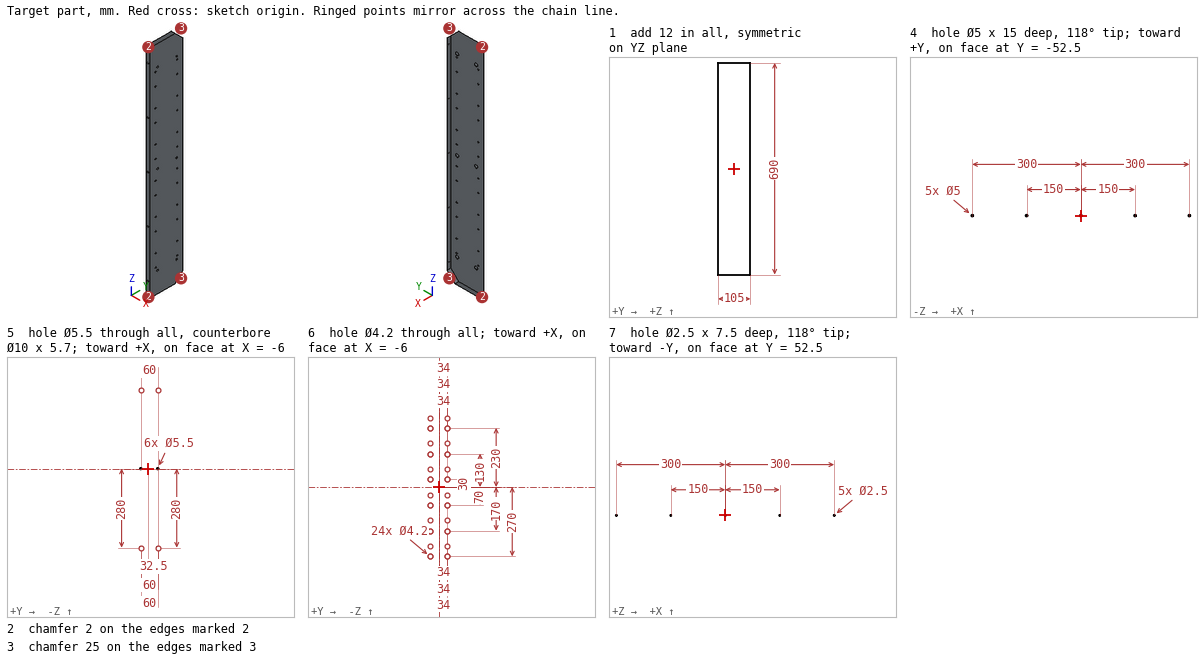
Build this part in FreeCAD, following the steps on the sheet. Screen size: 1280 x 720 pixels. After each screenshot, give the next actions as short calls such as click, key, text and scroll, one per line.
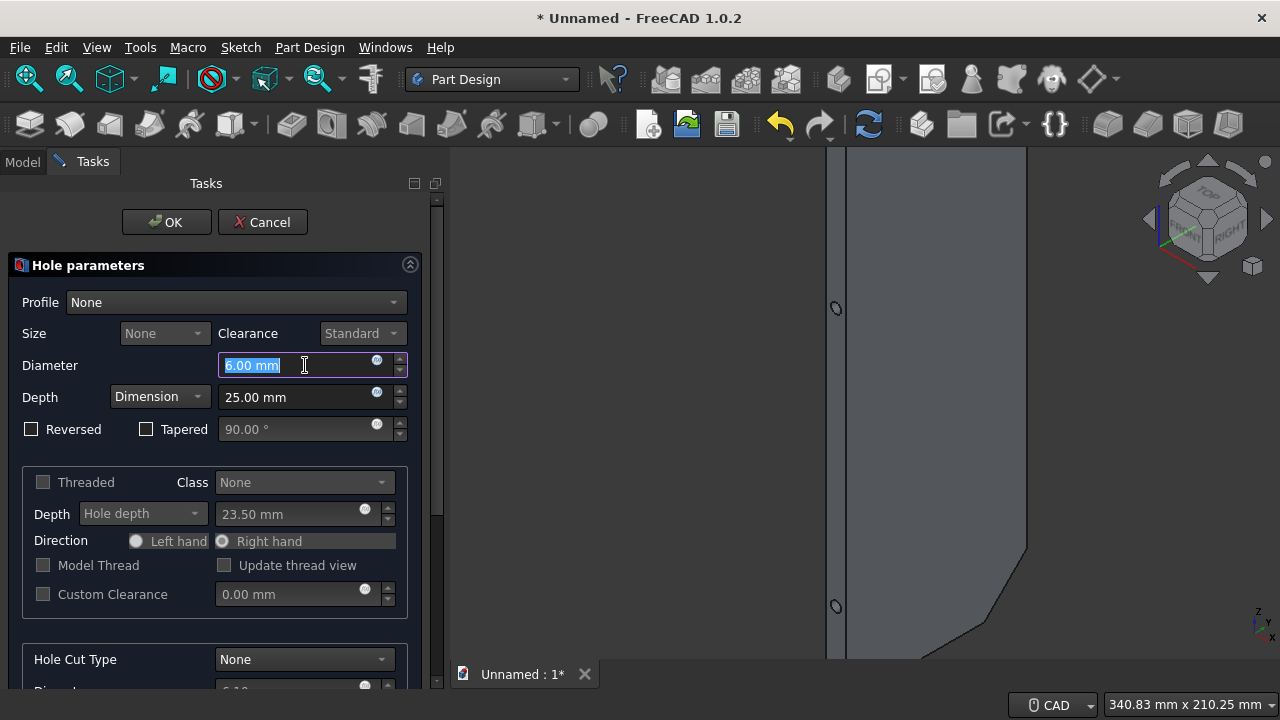
text(5)
key(Tab)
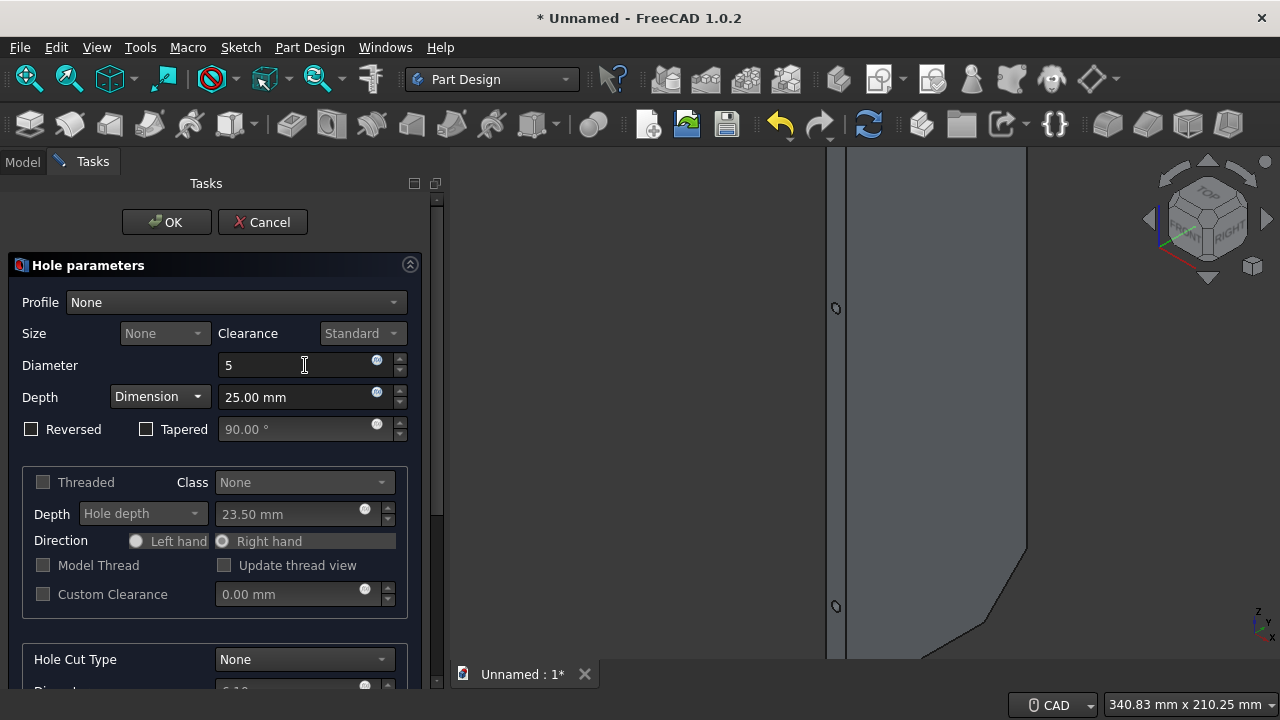
triple_click(305, 397)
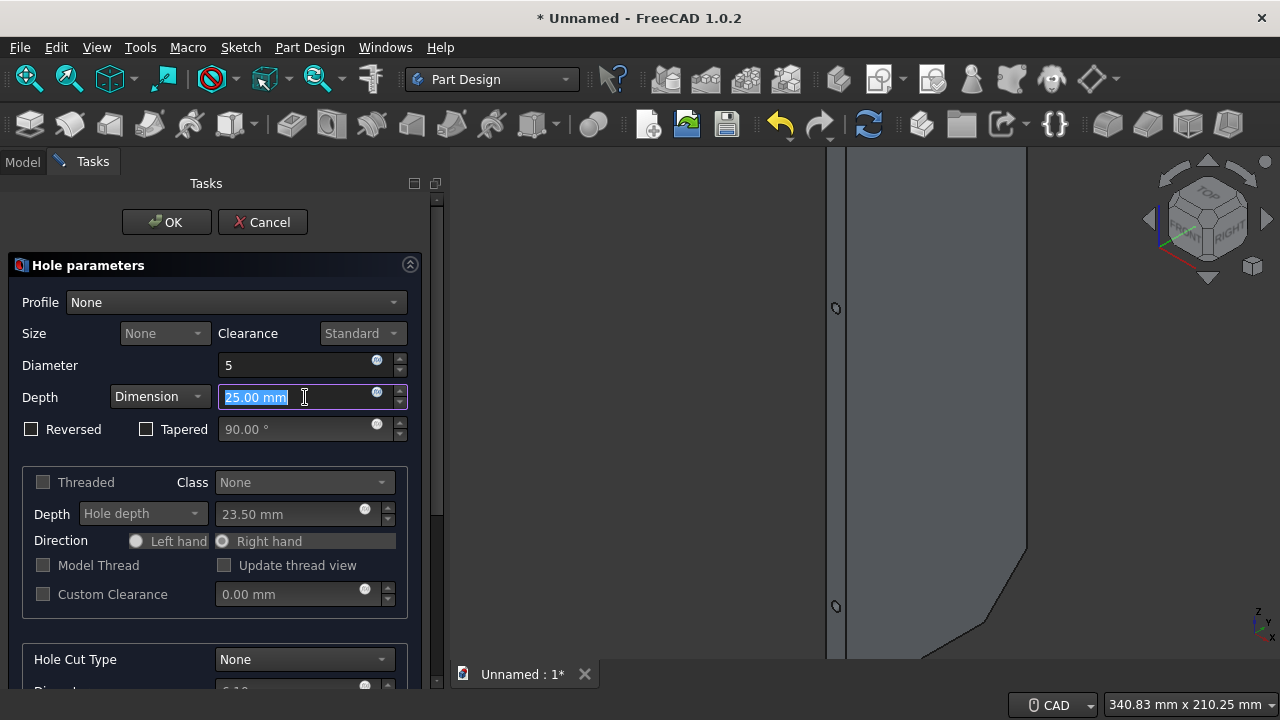
text(15)
key(Tab)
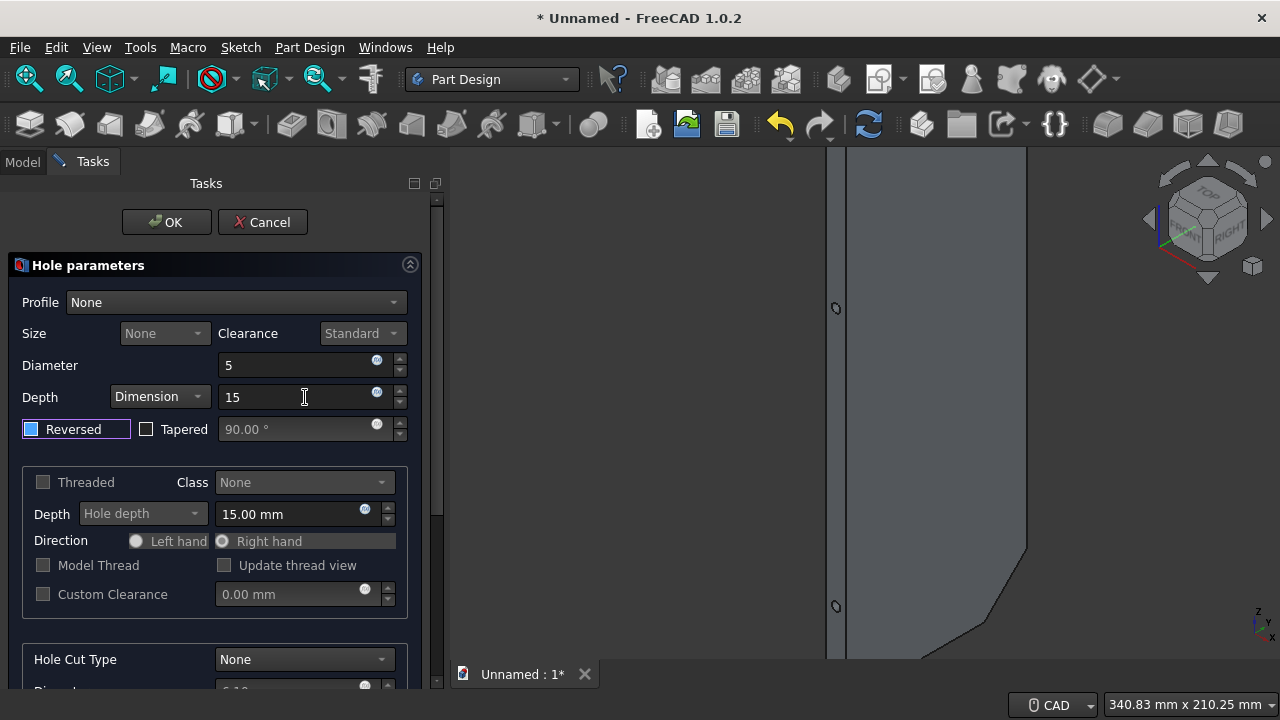
click(167, 222)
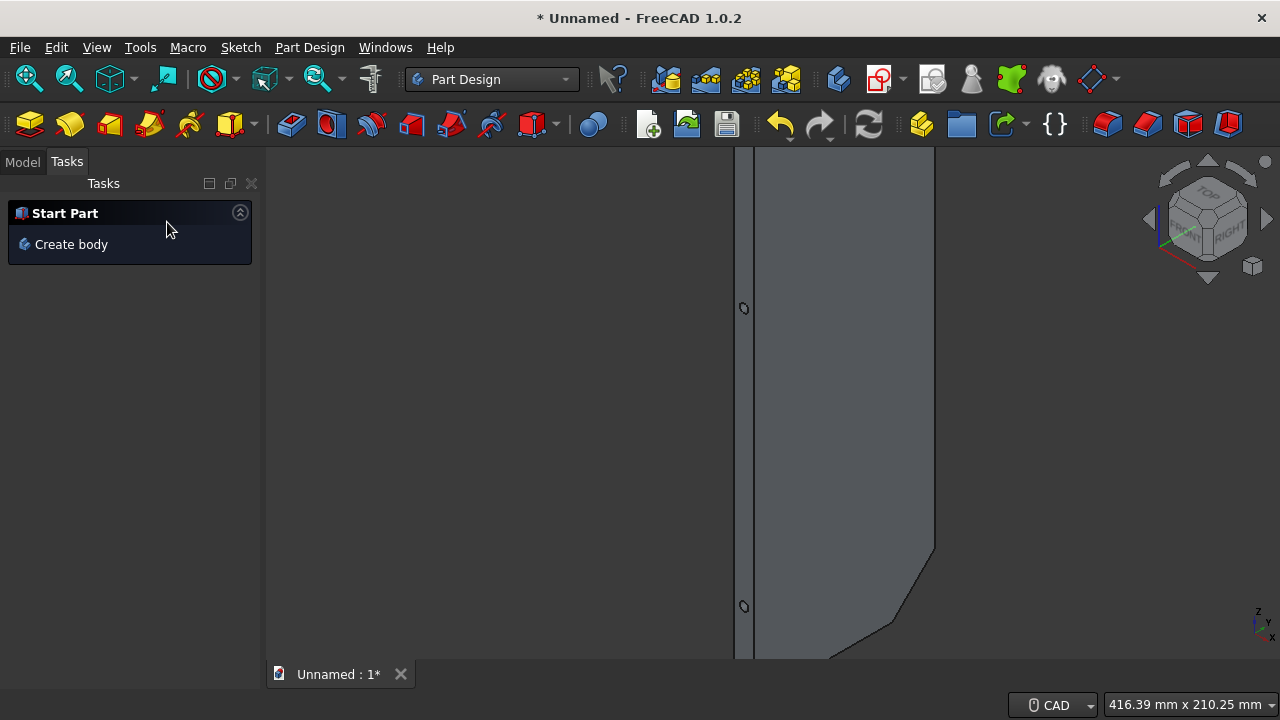
click(30, 80)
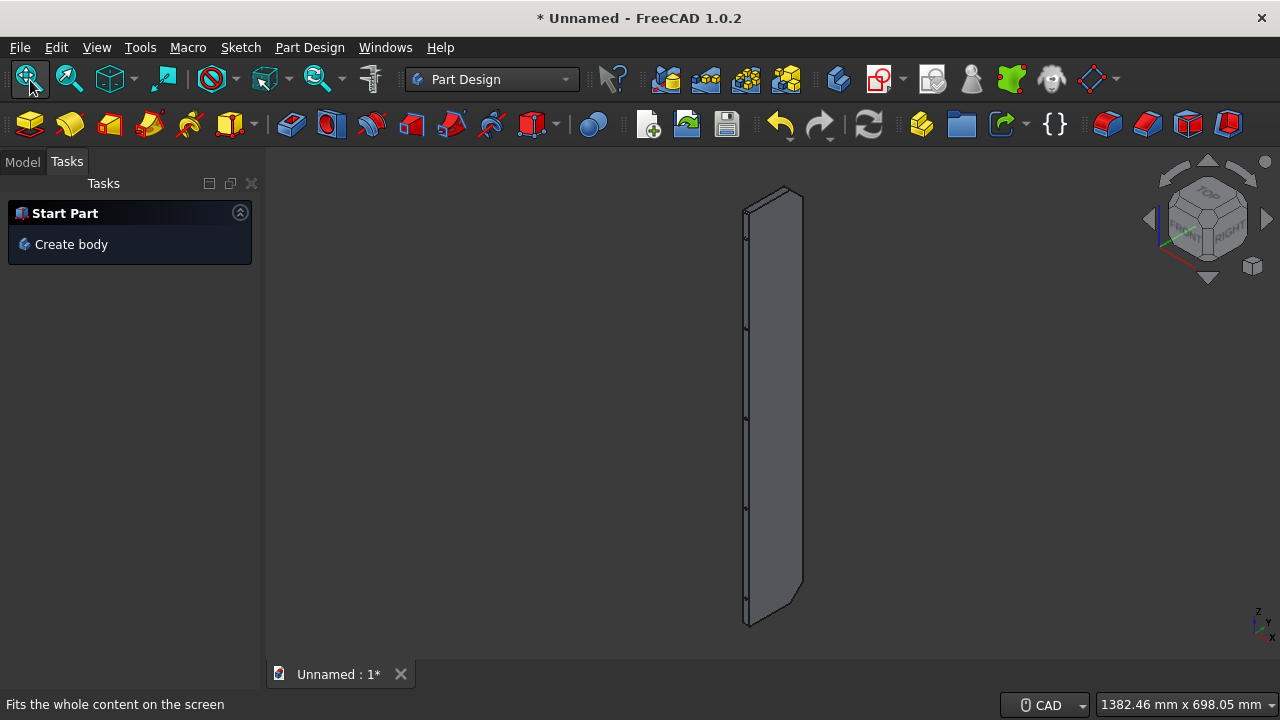
key(6)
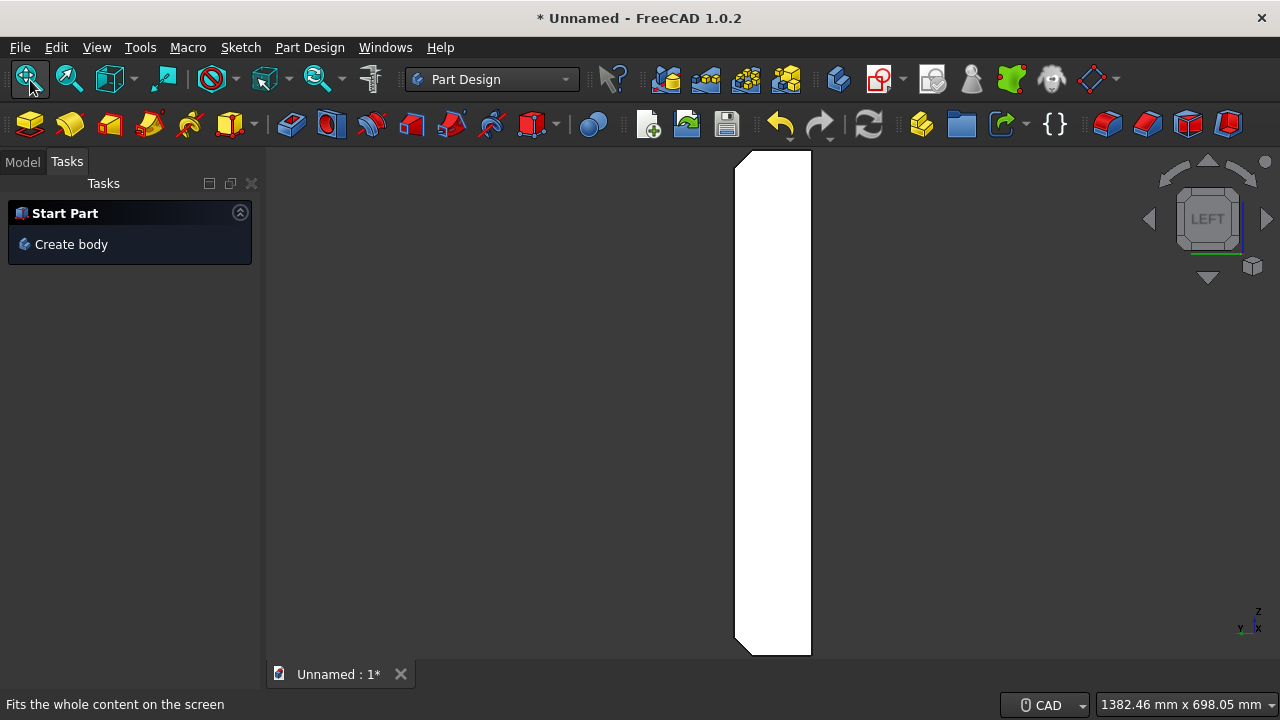
click(773, 547)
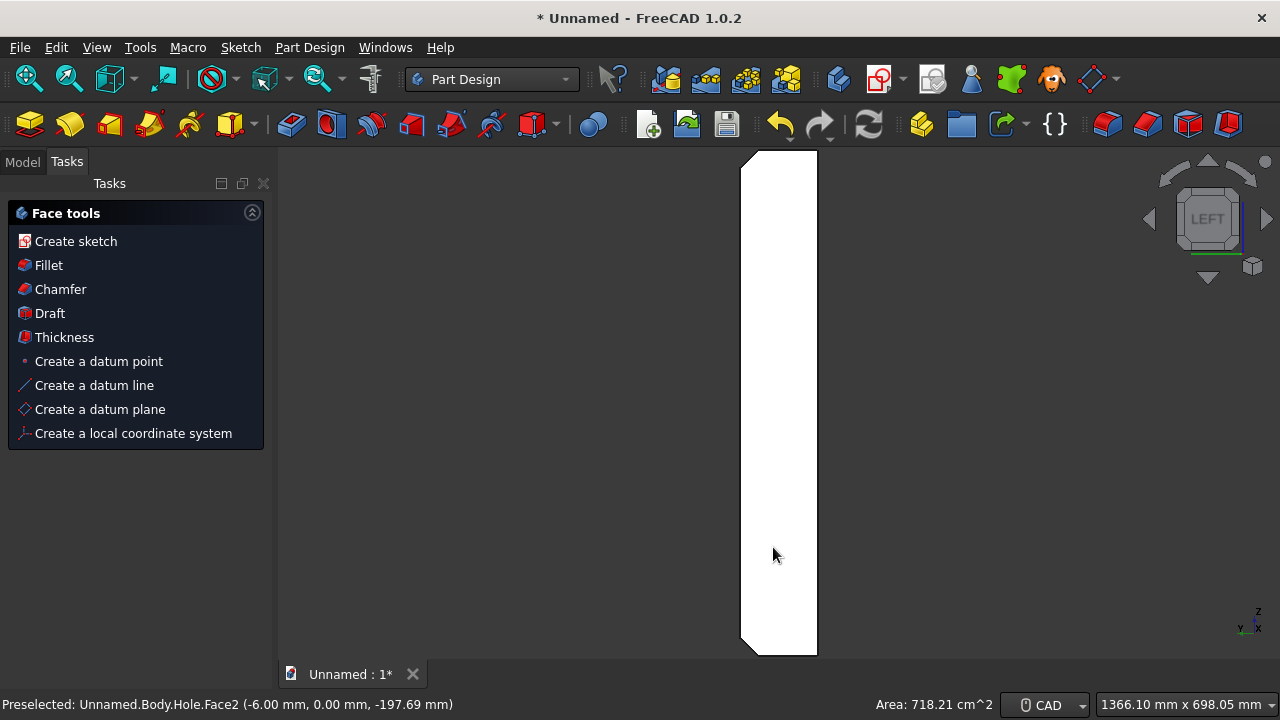
click(880, 80)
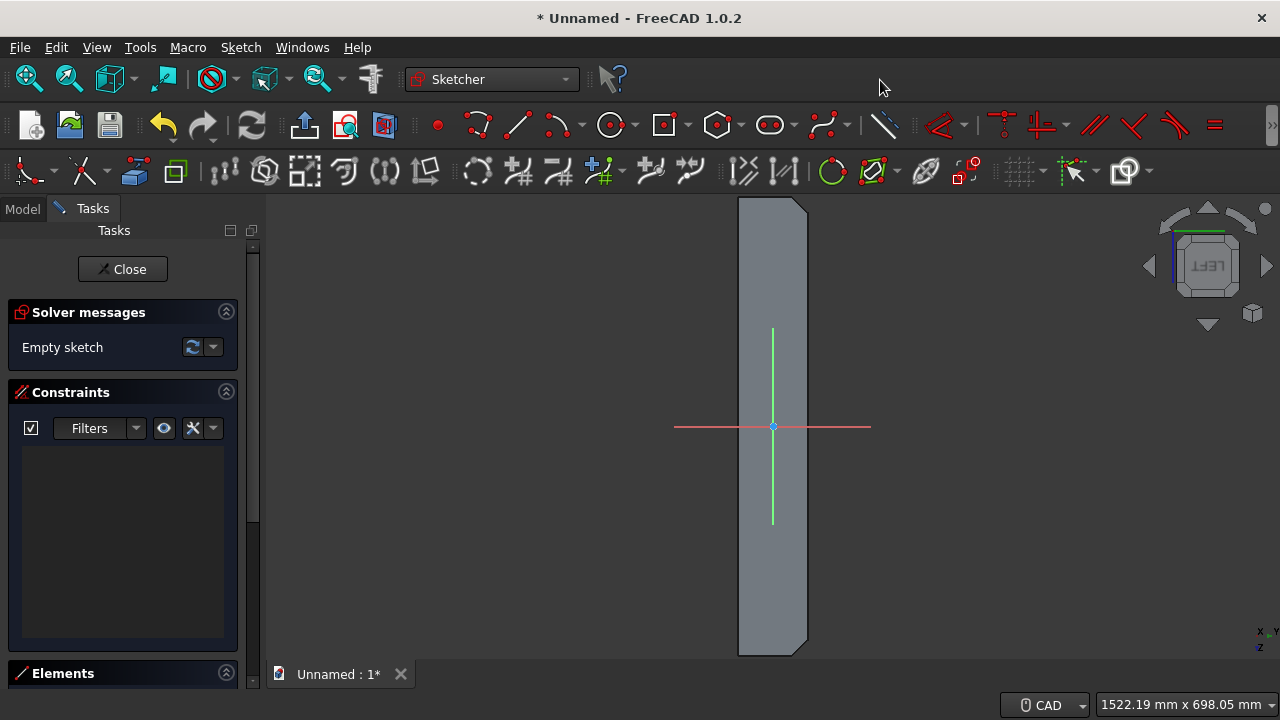
scroll(388, 427, down, 1)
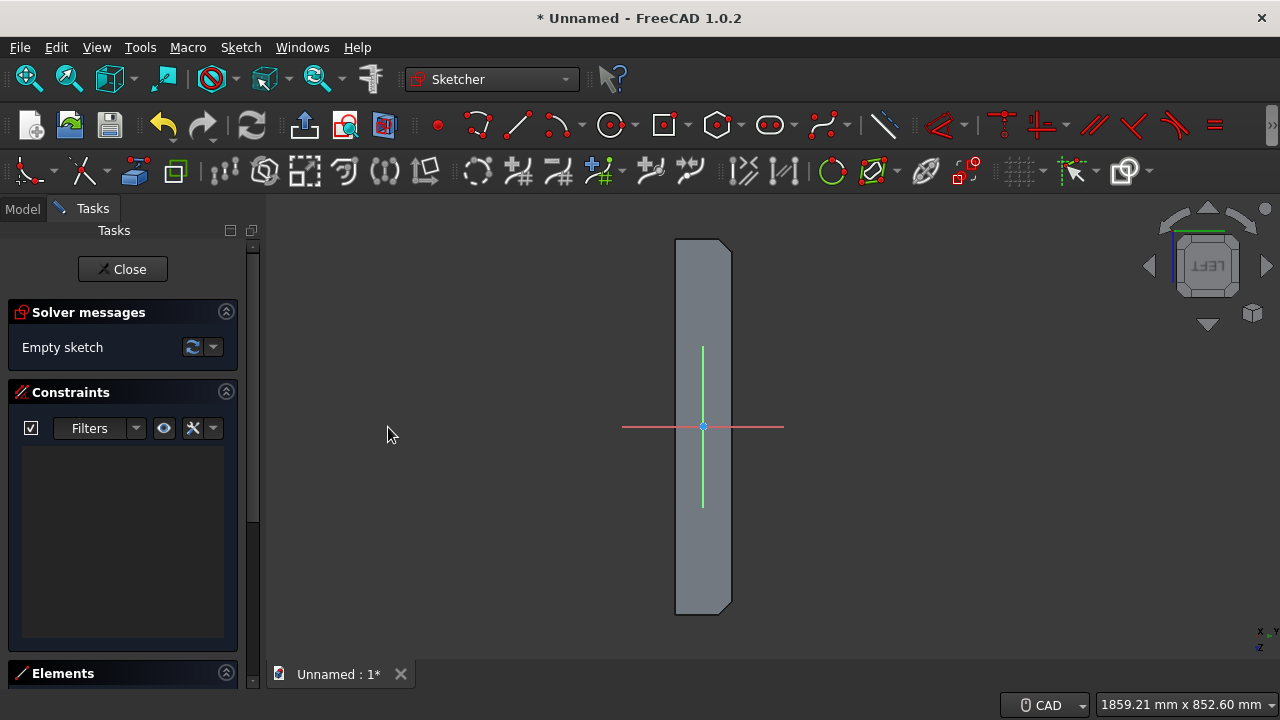
click(612, 126)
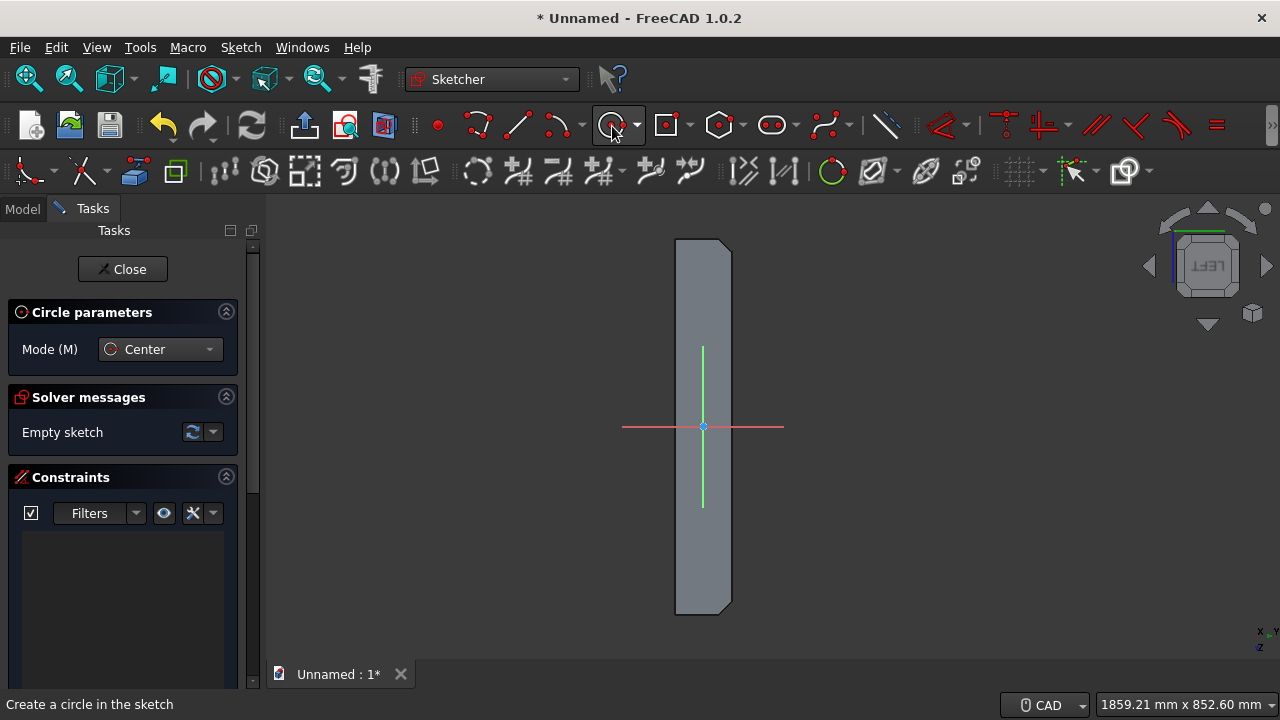
scroll(721, 579, up, 14)